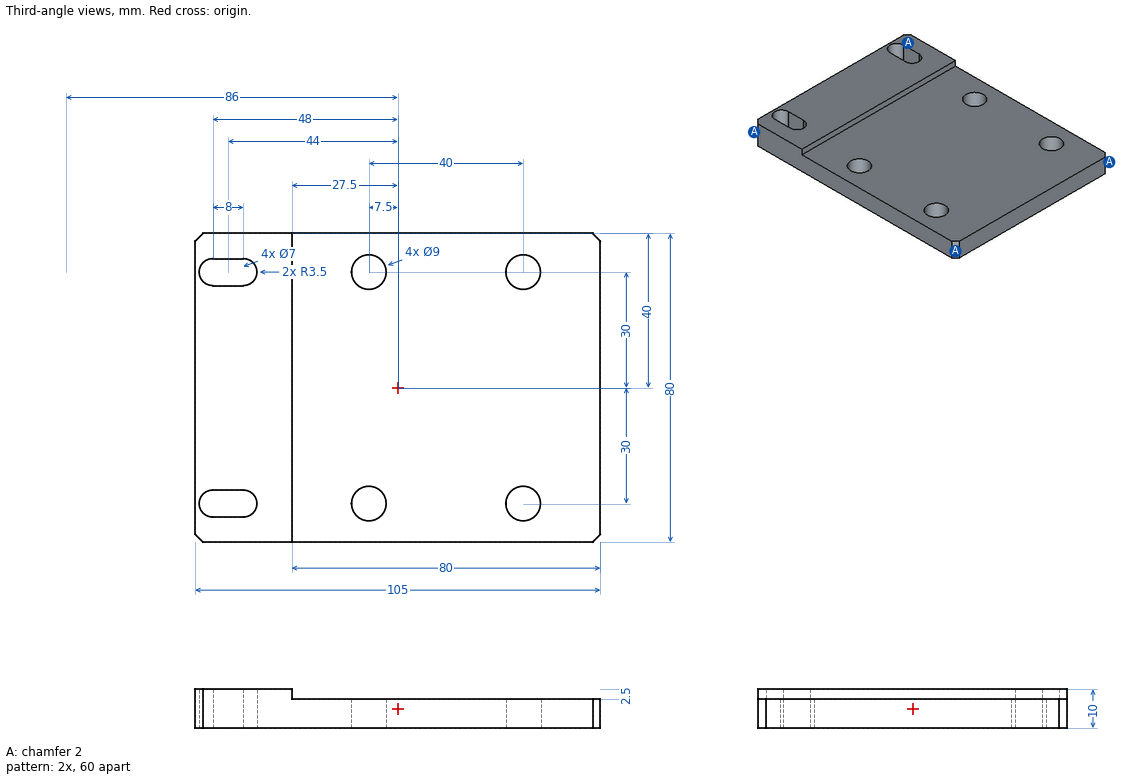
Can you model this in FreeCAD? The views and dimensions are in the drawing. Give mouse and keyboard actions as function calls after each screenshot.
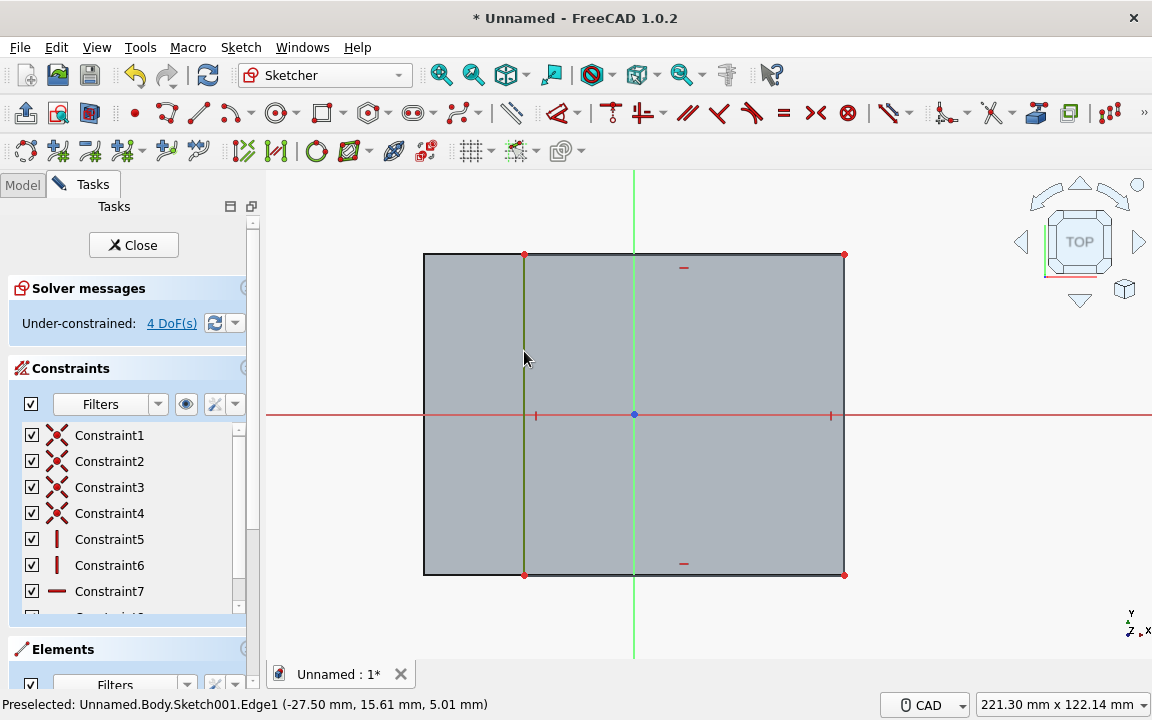
key(i)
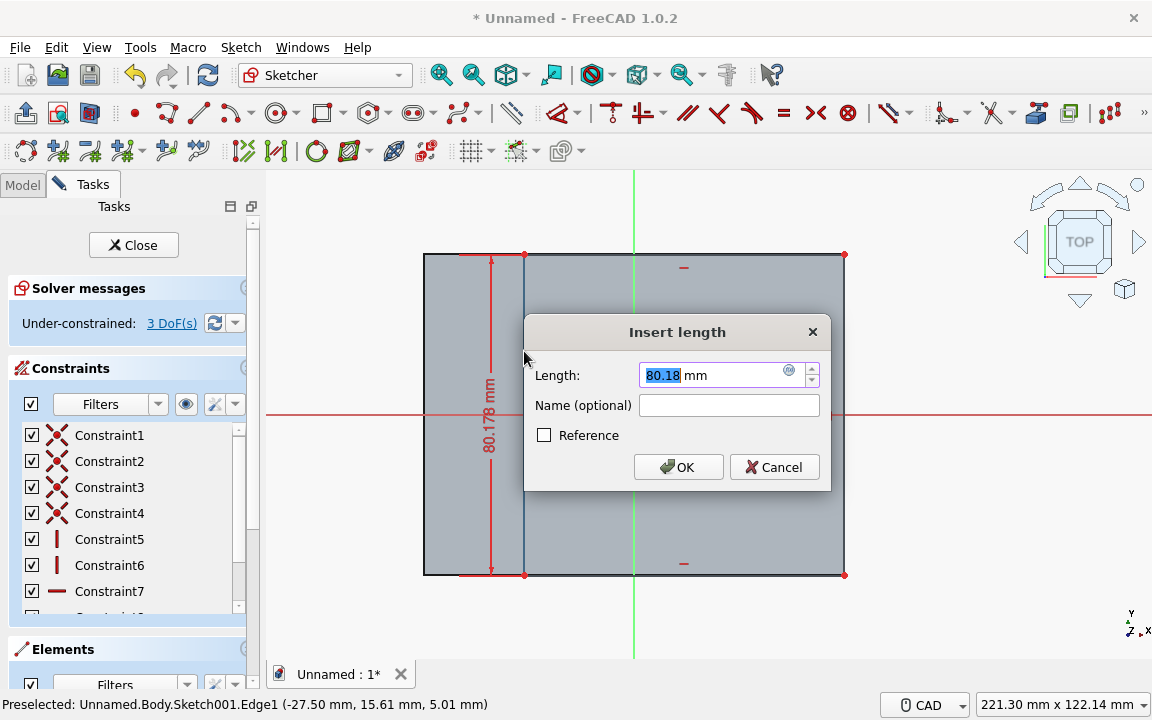
text(80)
key(Return)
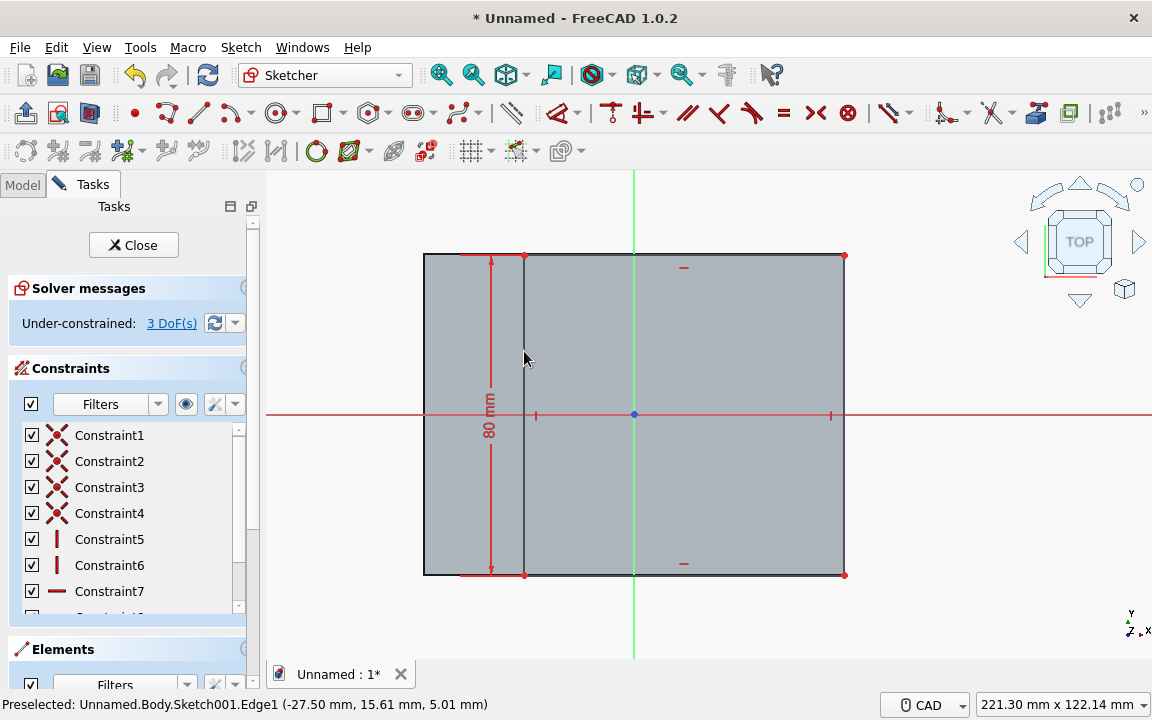
click(620, 576)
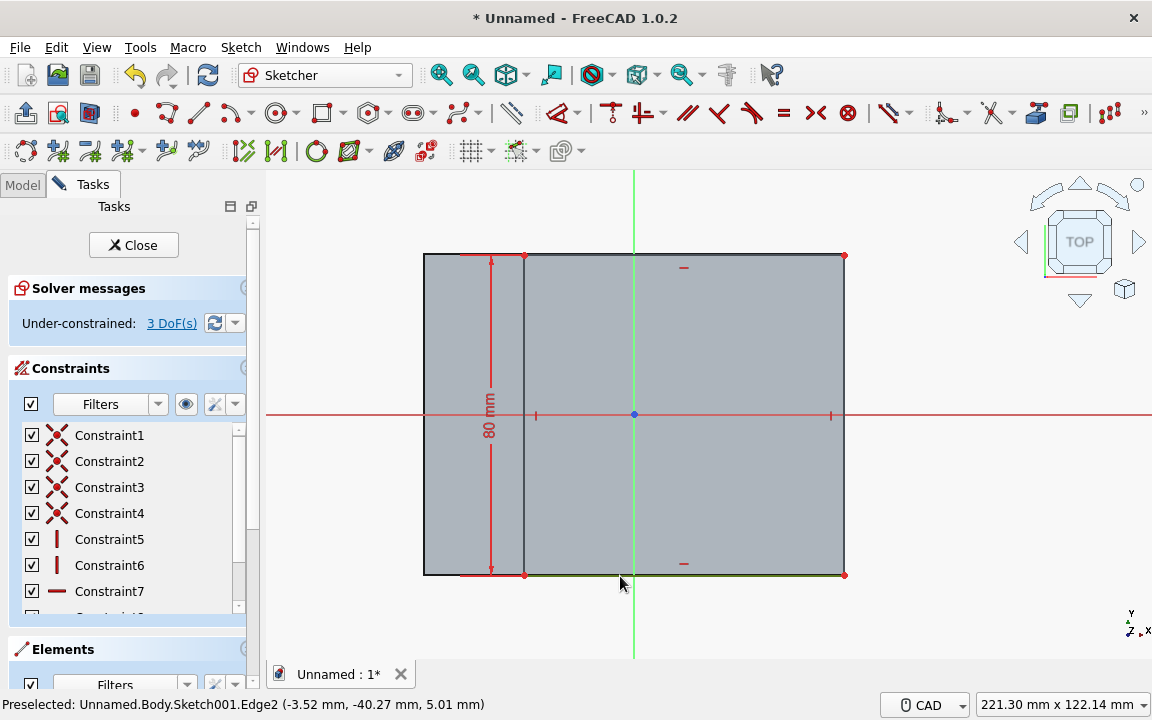
click(580, 114)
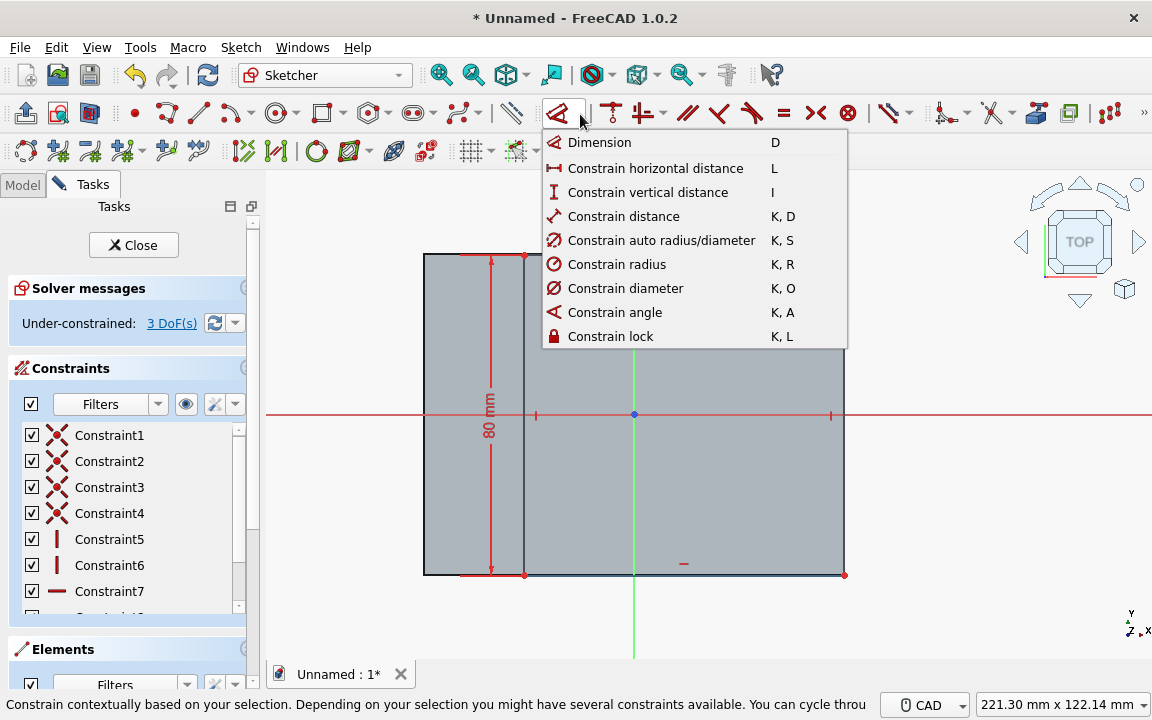
click(695, 168)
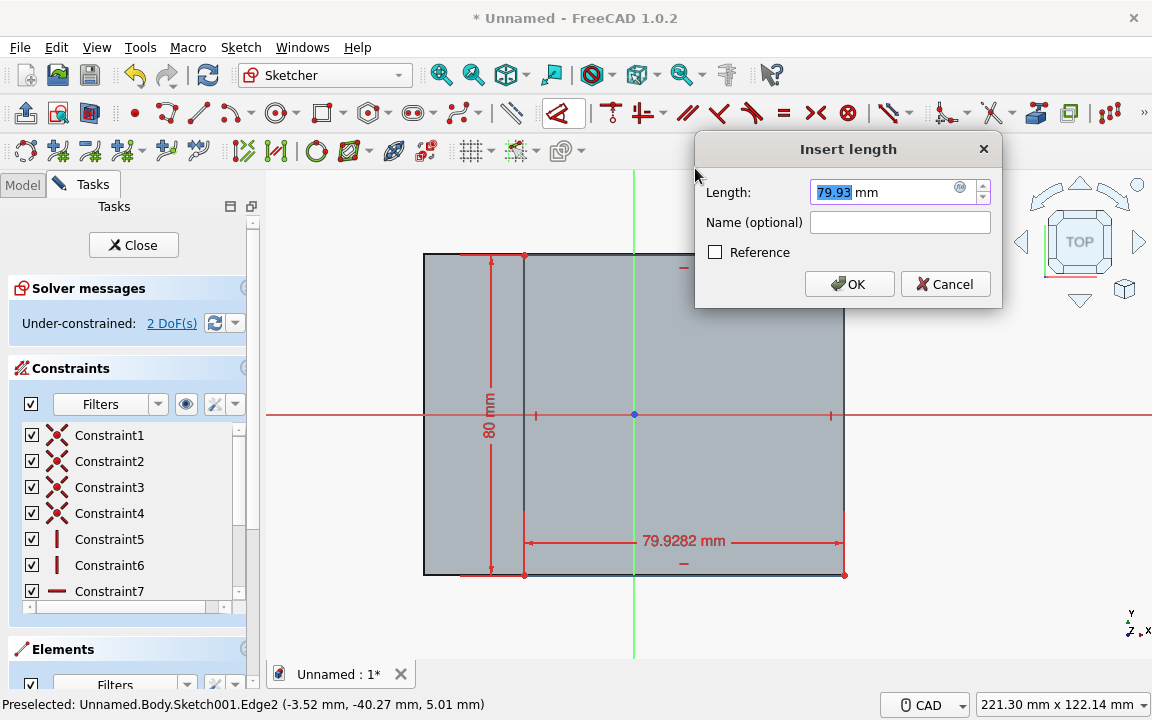
text(80)
key(Return)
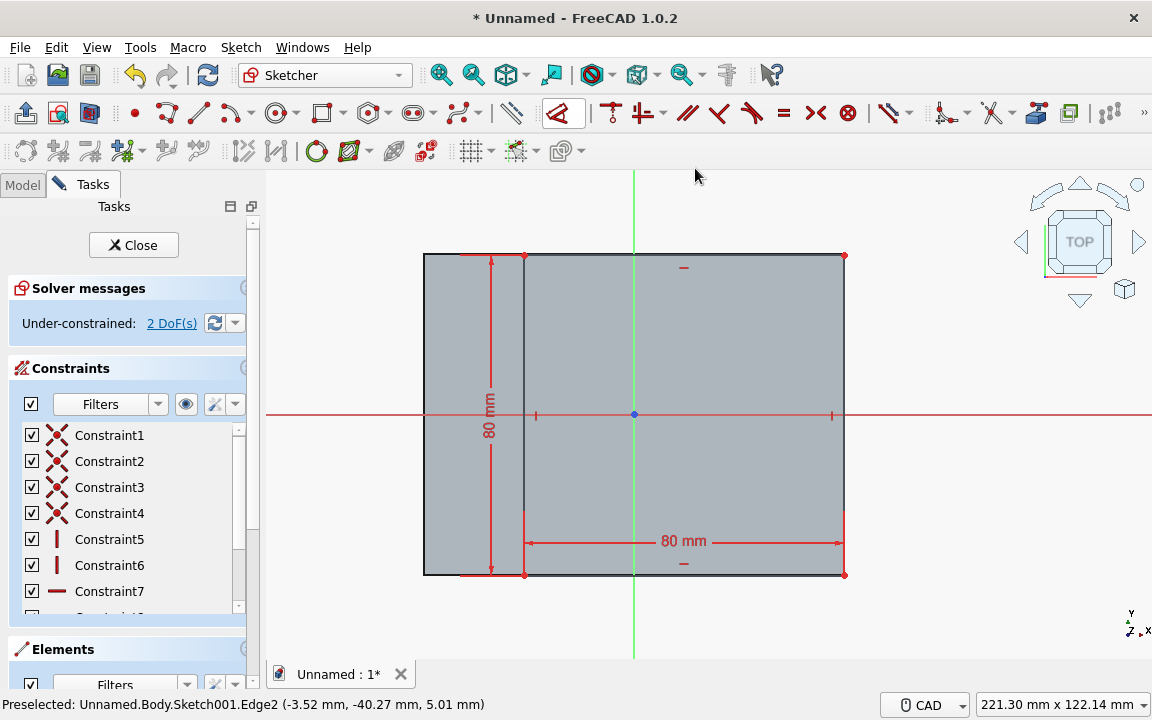
click(524, 255)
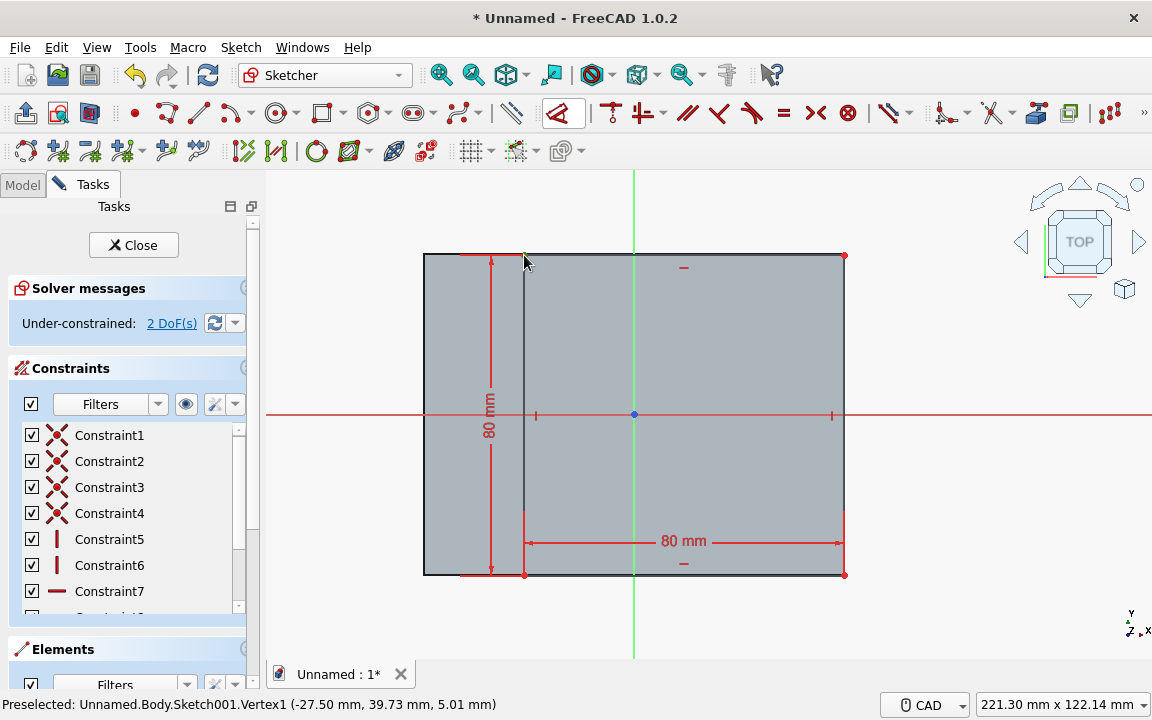
key(i)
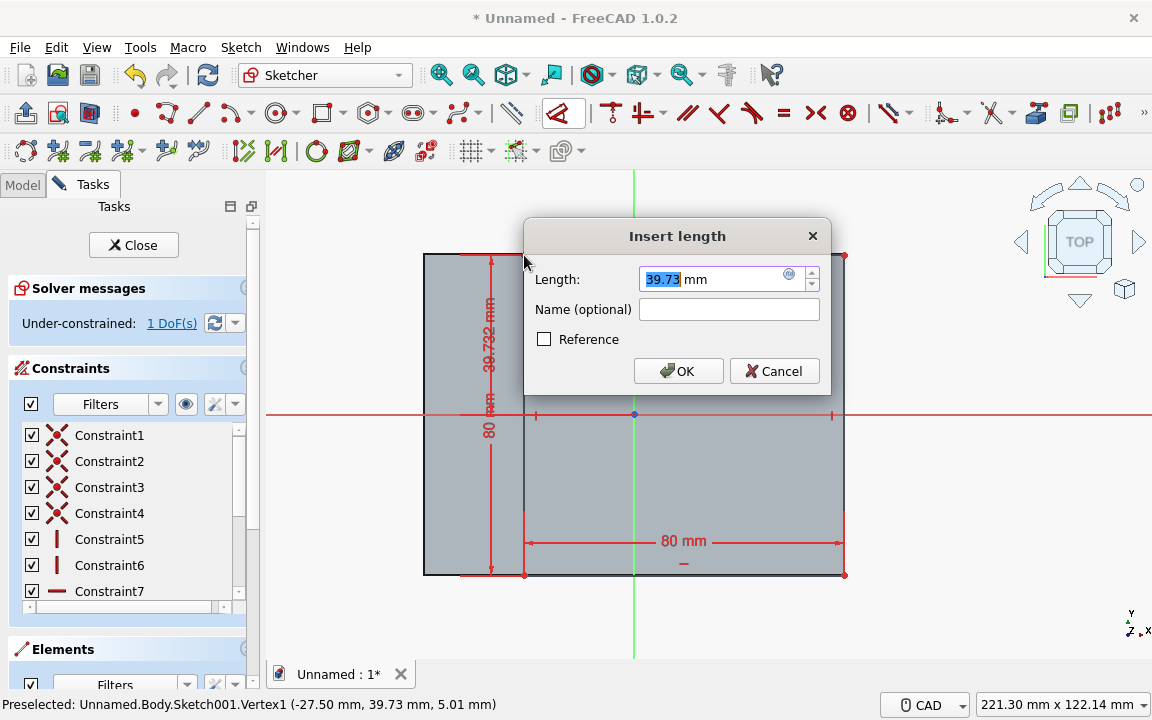
text(40)
key(Return)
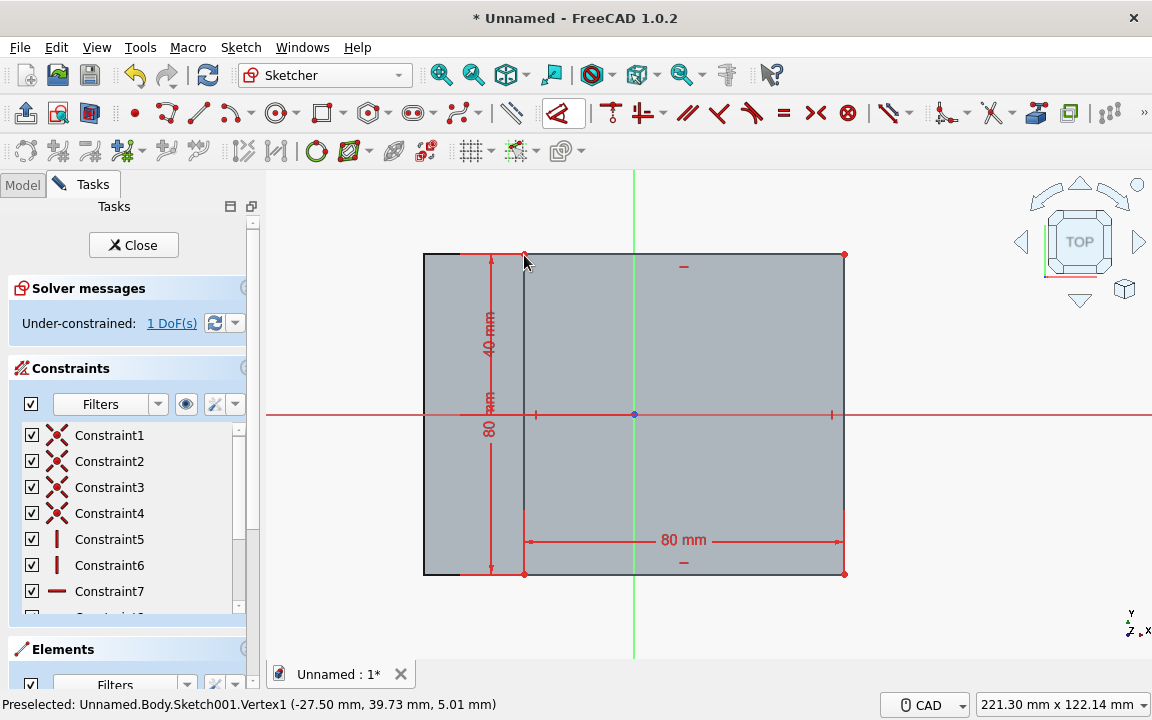
click(524, 254)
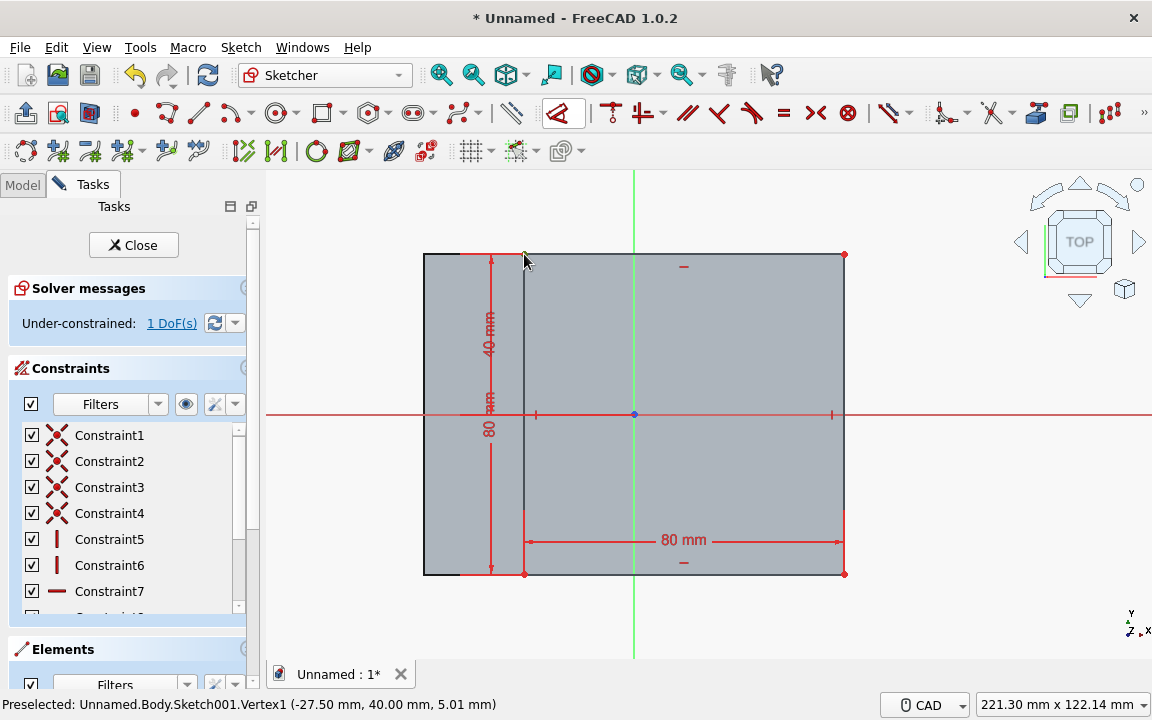
key(l)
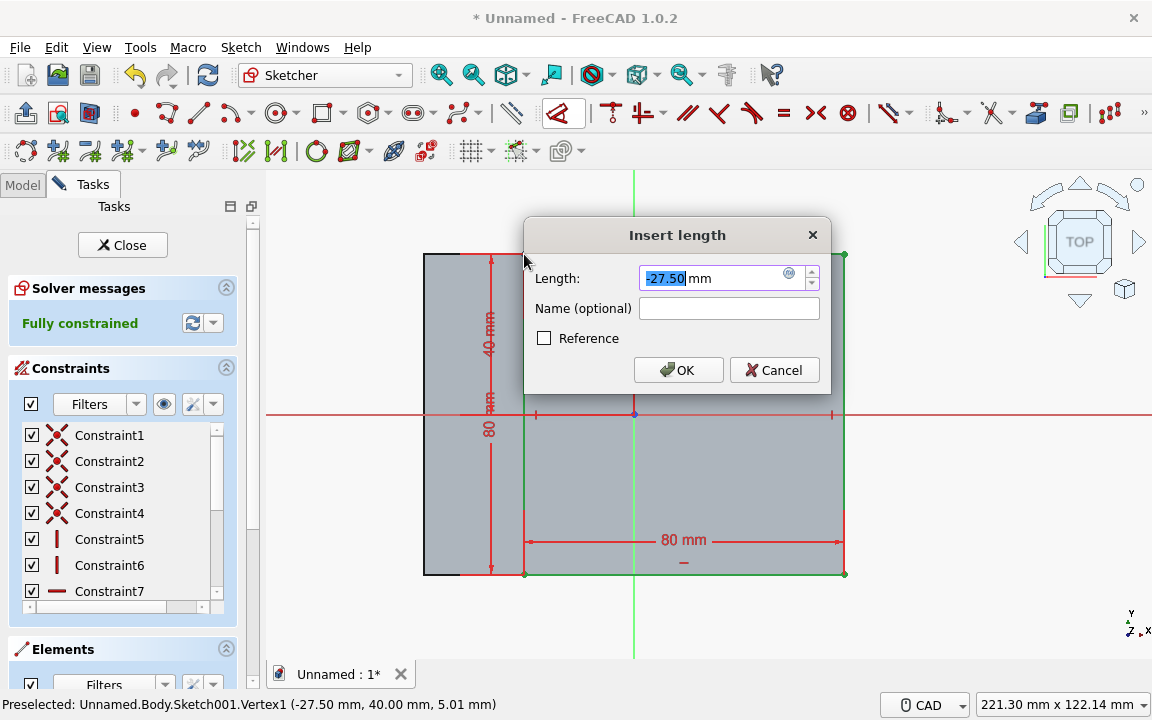
text(-27.5)
key(Return)